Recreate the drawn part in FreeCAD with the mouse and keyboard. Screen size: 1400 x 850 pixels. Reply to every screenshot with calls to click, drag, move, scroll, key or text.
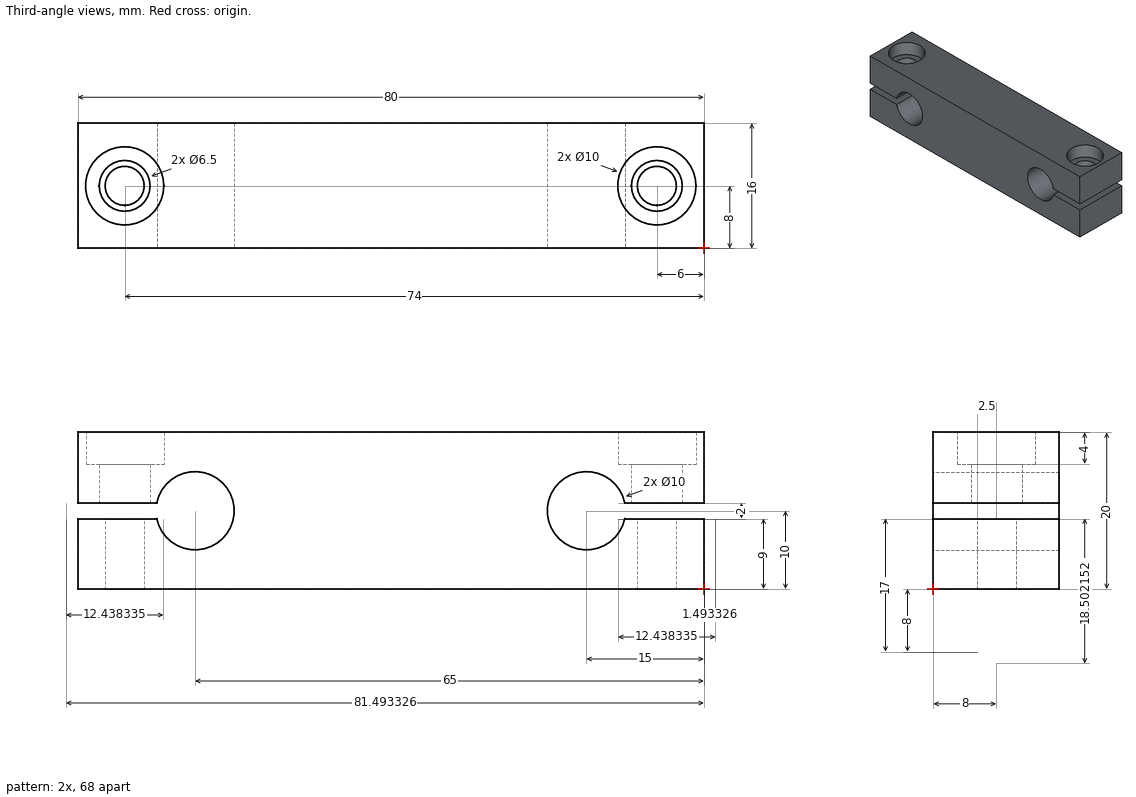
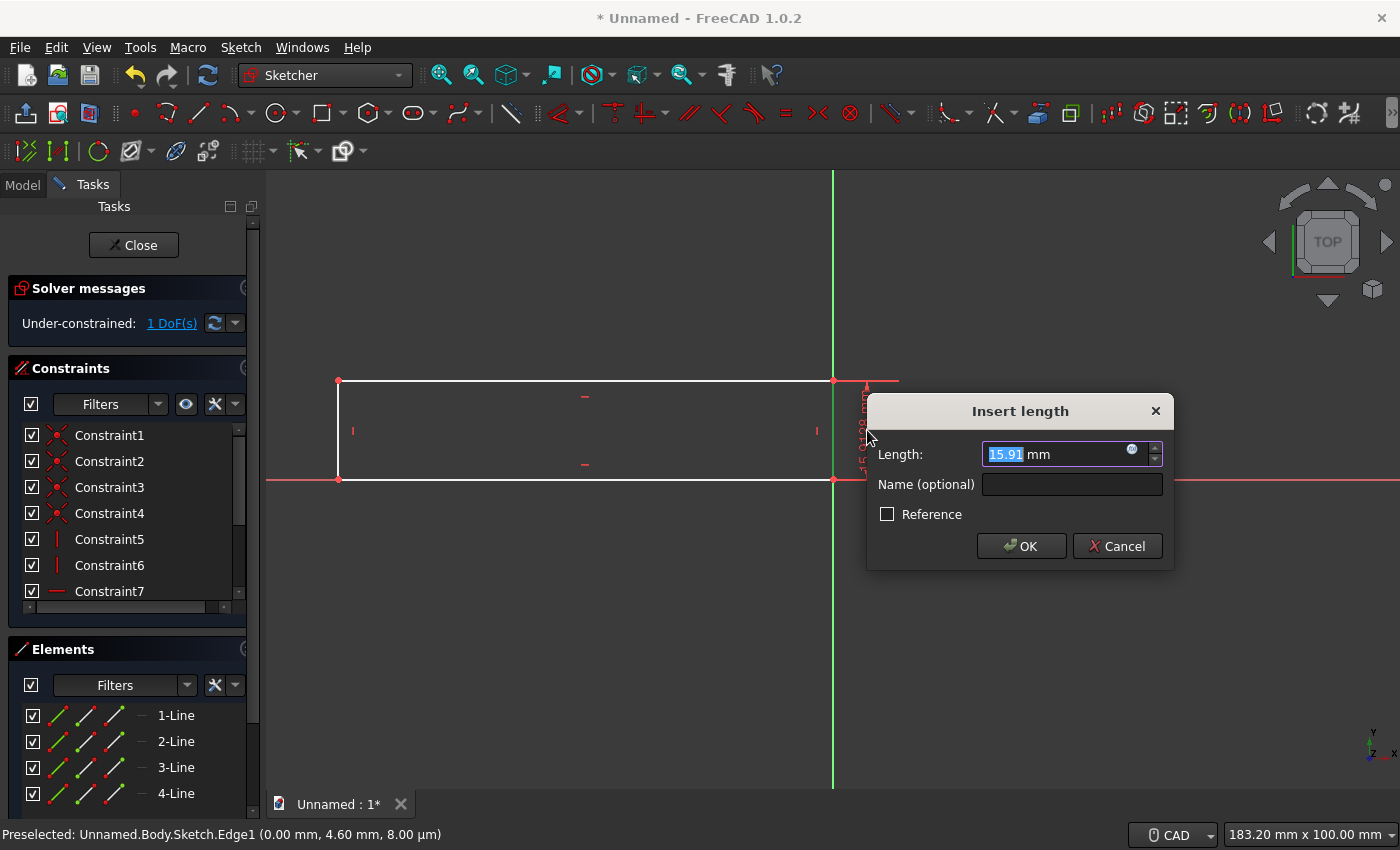
text(16)
key(Return)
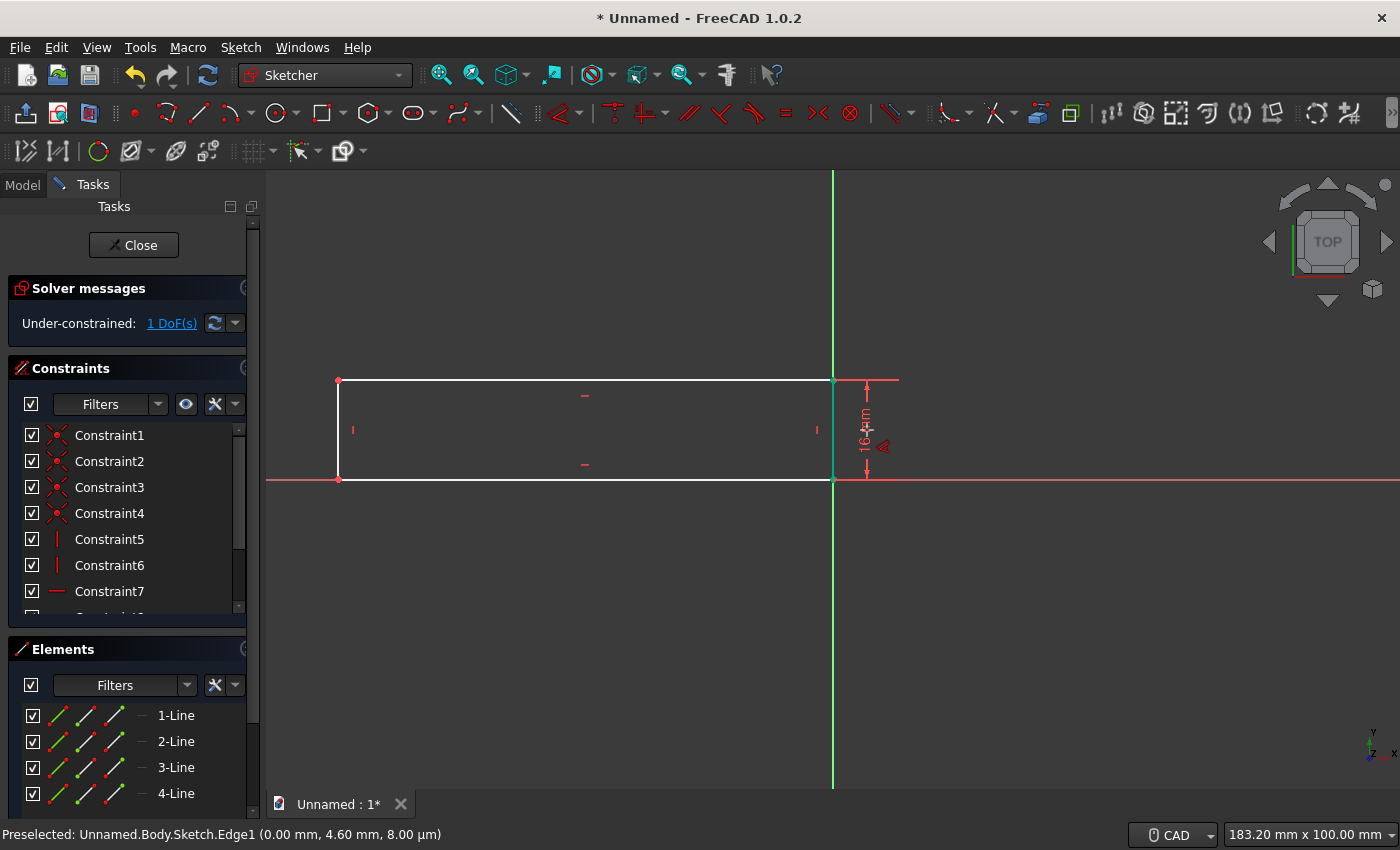
click(684, 380)
click(585, 346)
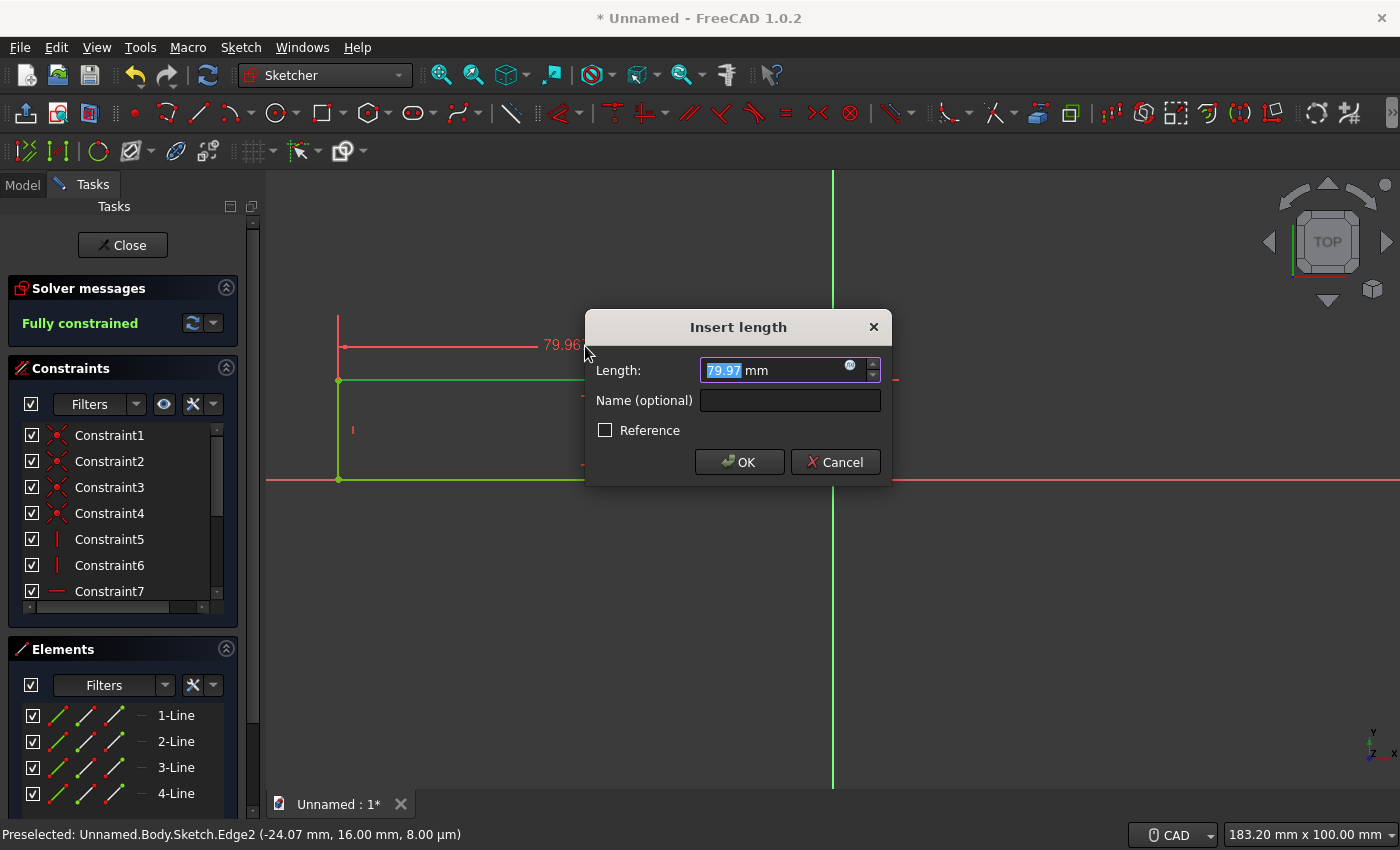
text(80)
key(Return)
key(Escape)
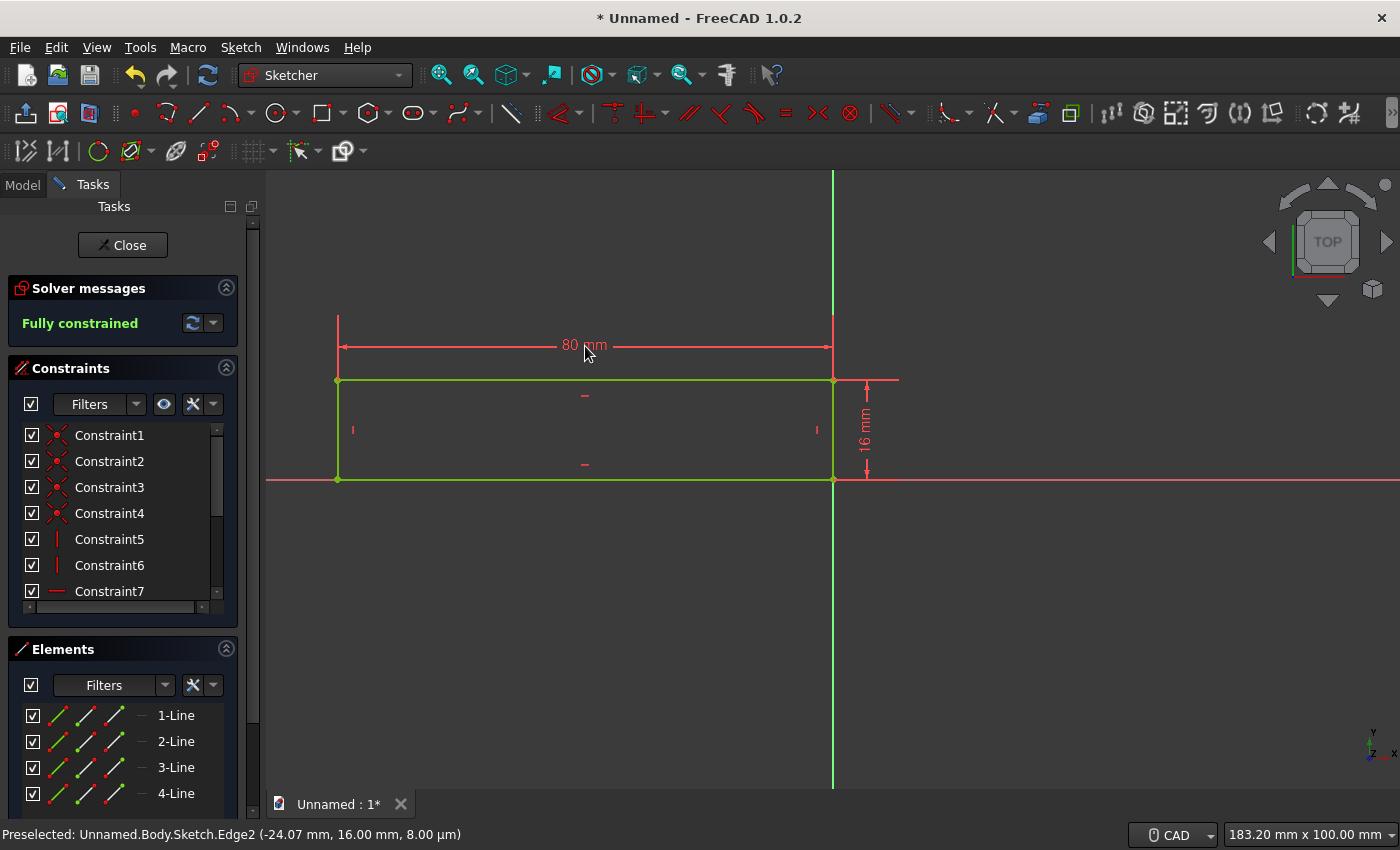
click(123, 245)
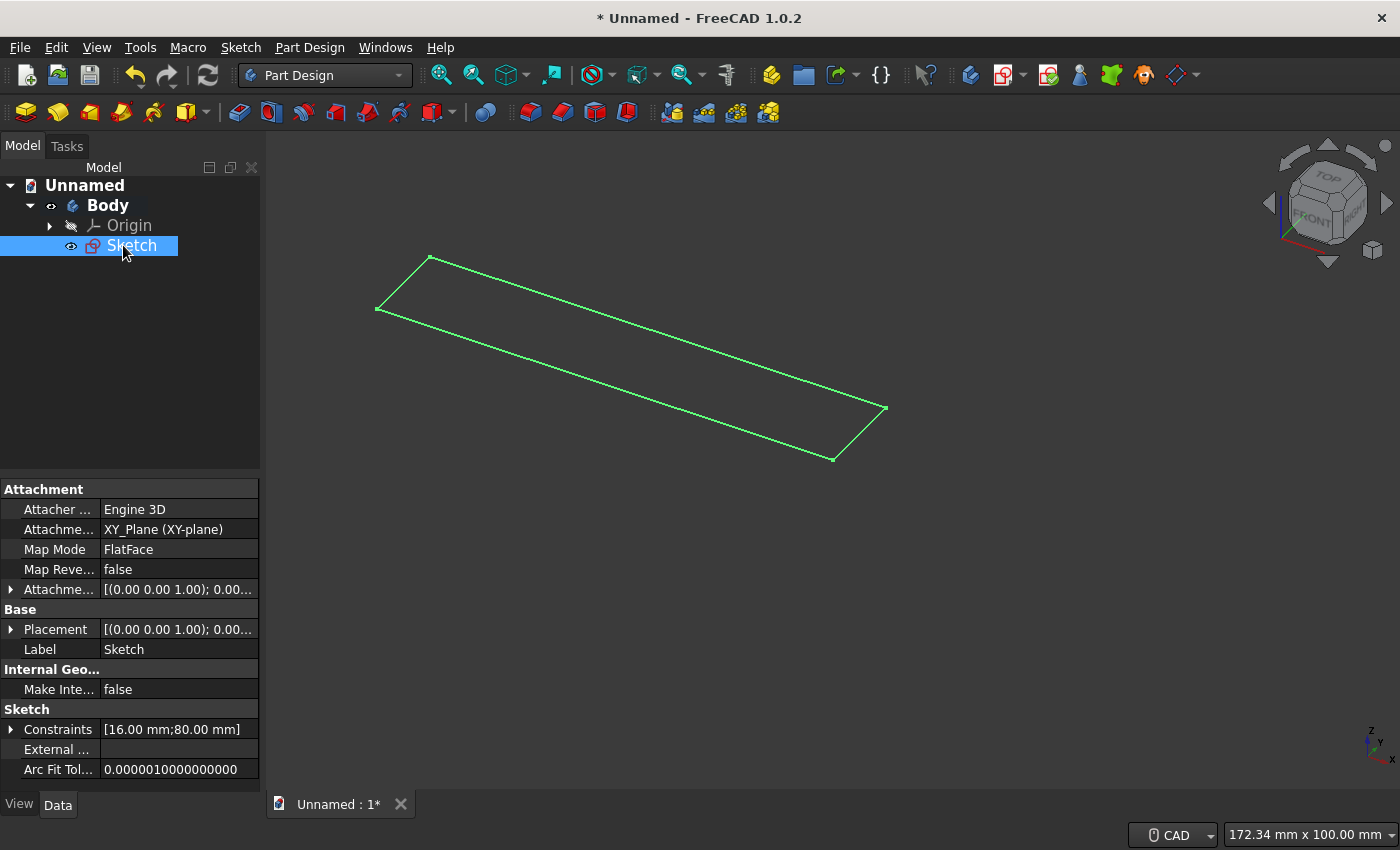
click(26, 112)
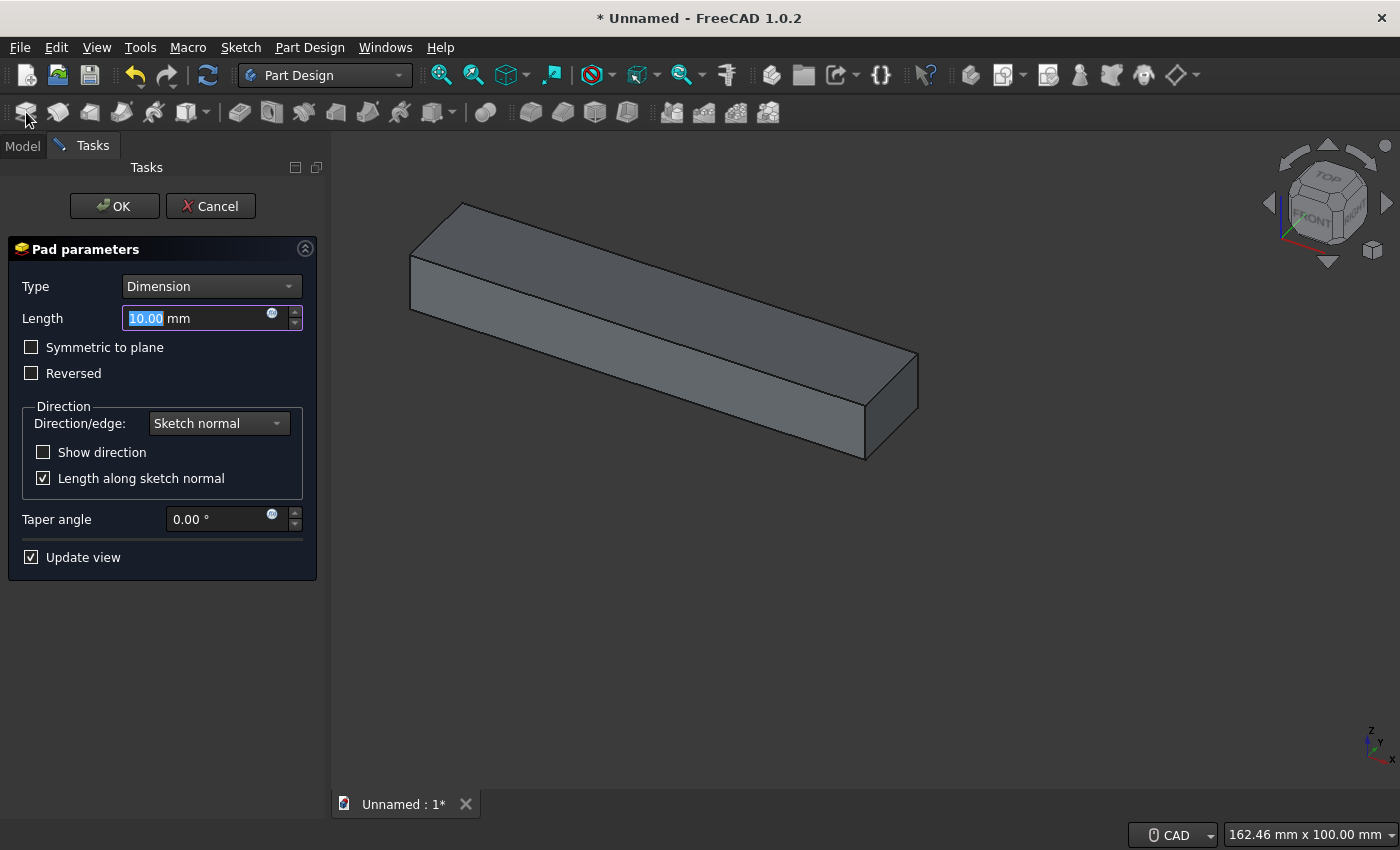
text(20)
key(Tab)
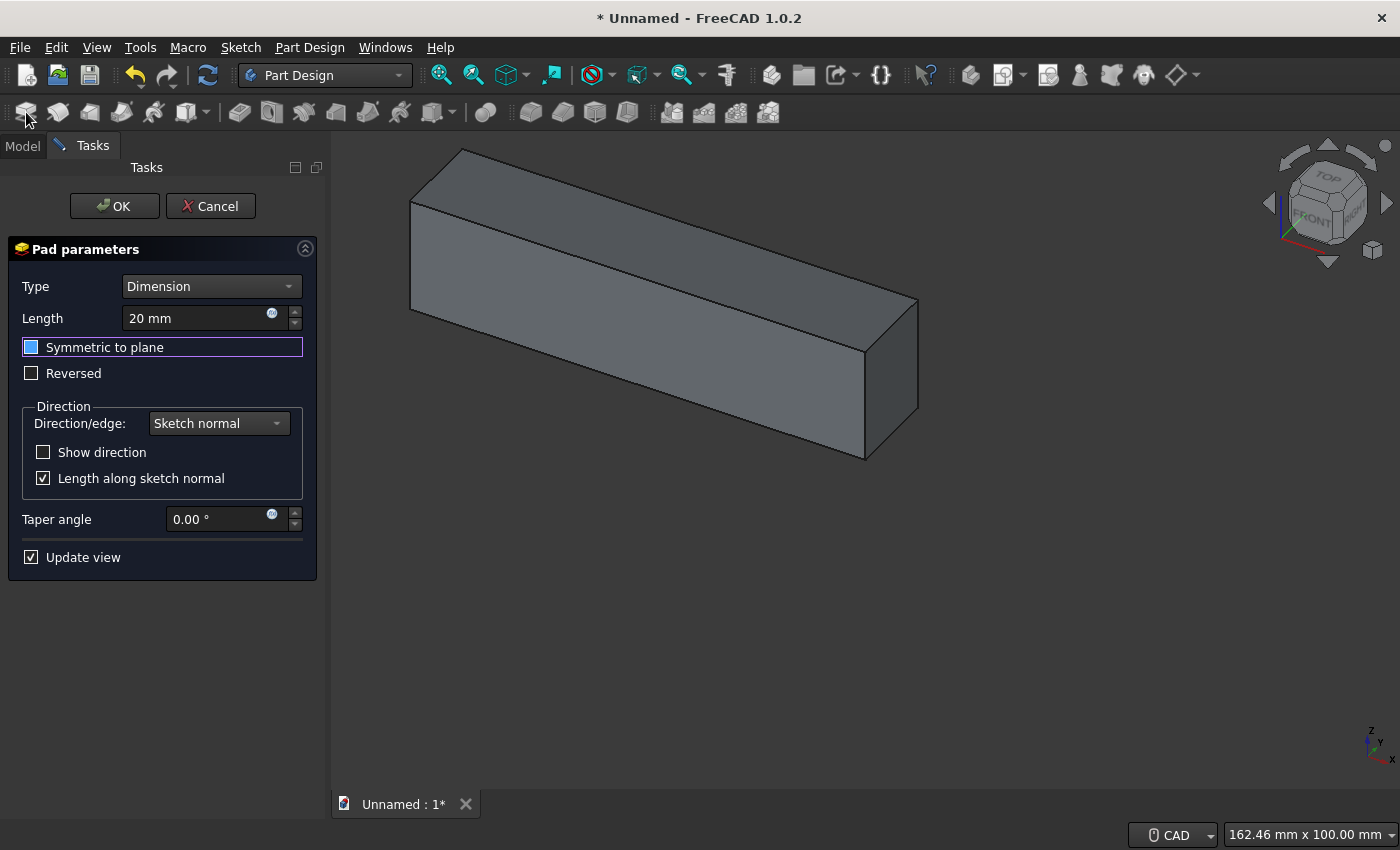
click(115, 206)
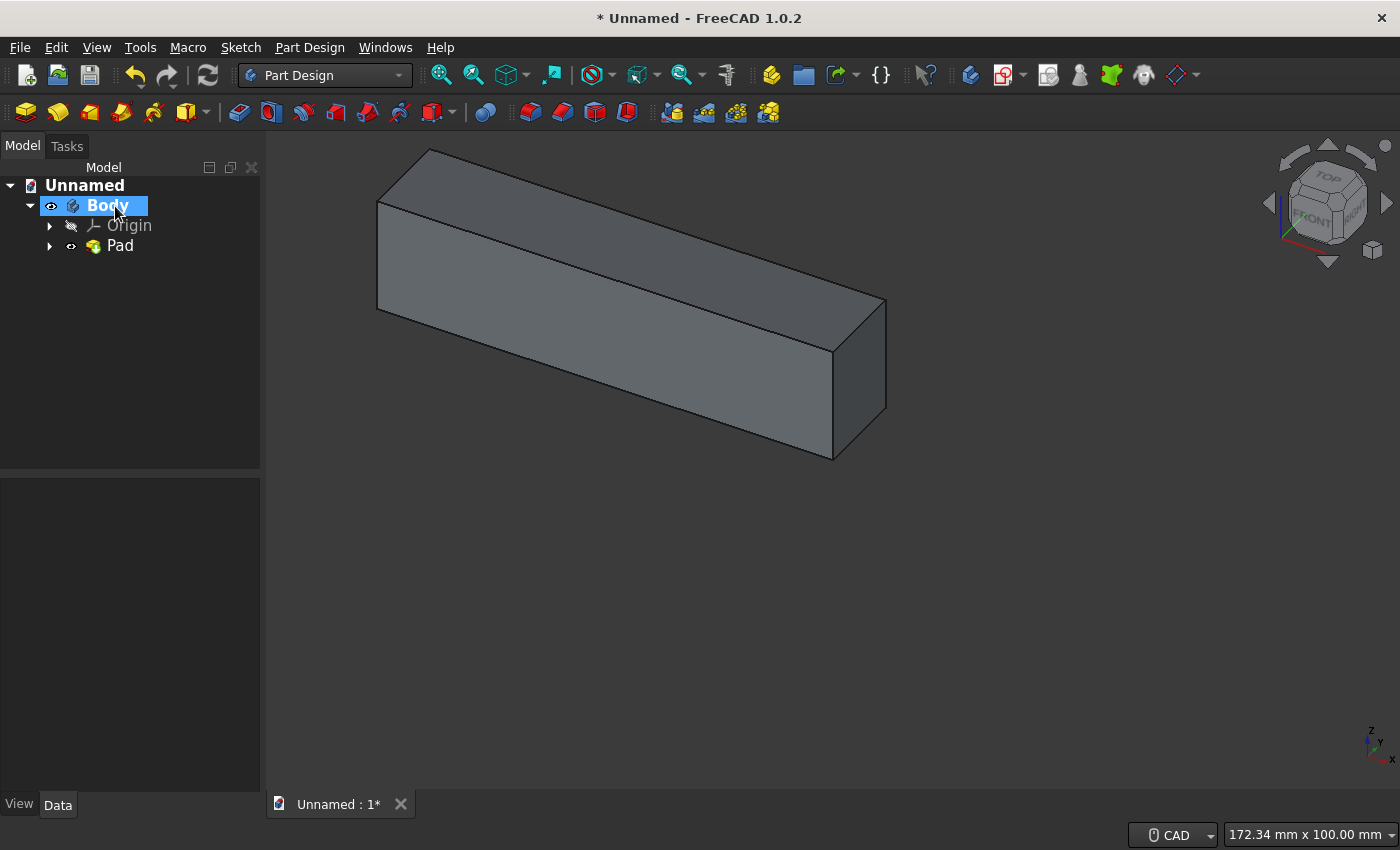
click(1004, 76)